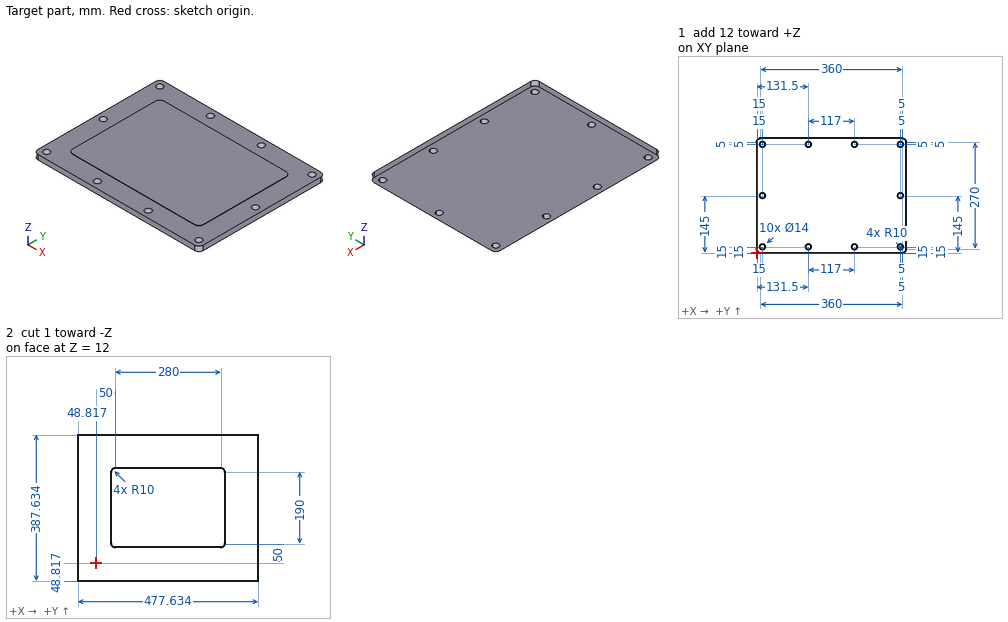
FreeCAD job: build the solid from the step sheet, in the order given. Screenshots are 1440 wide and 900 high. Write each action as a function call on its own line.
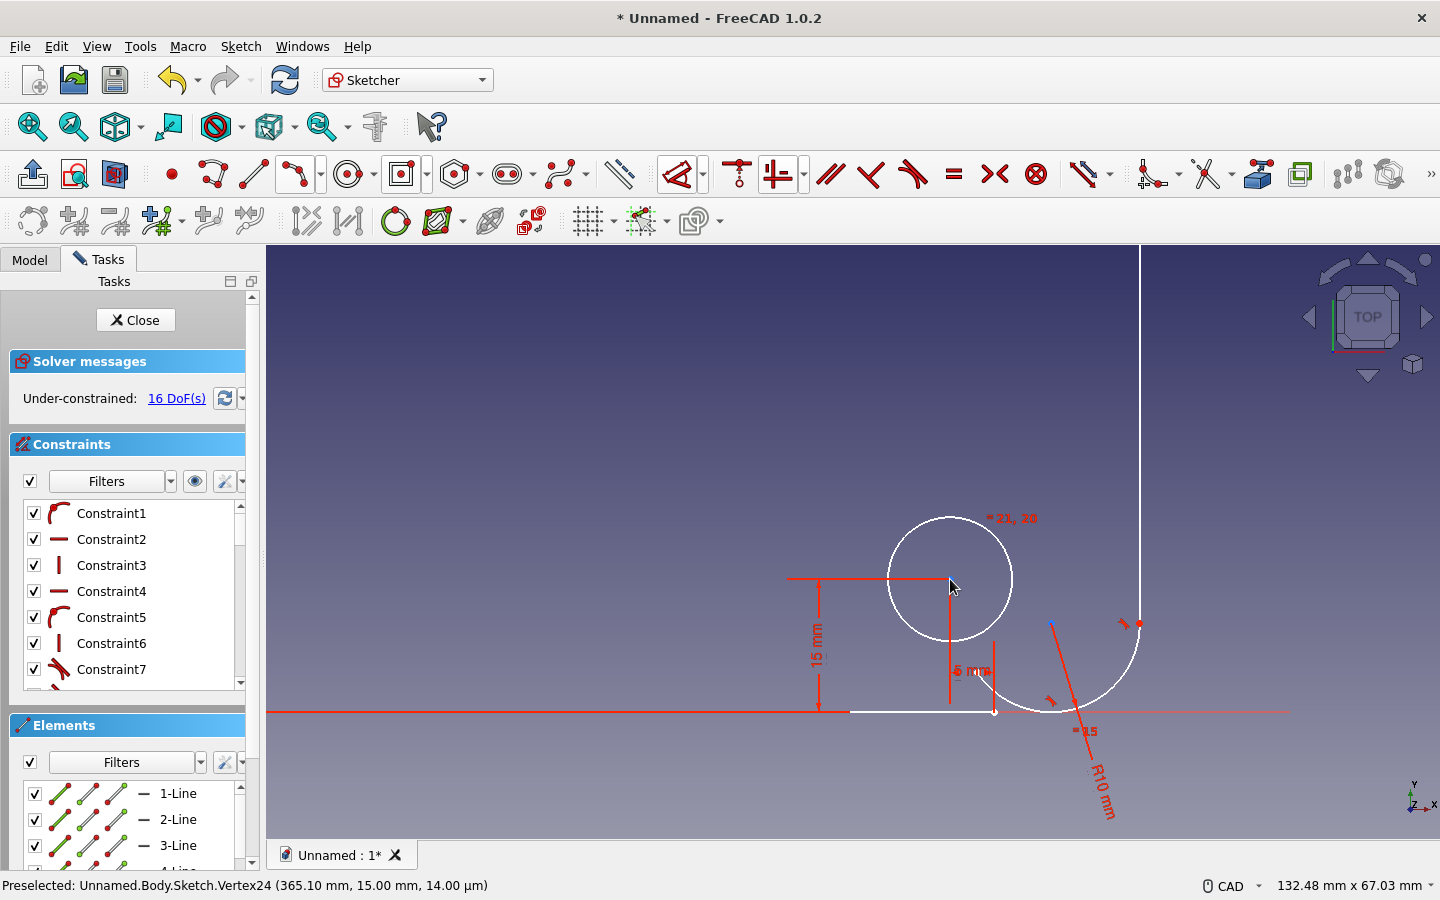
click(977, 673)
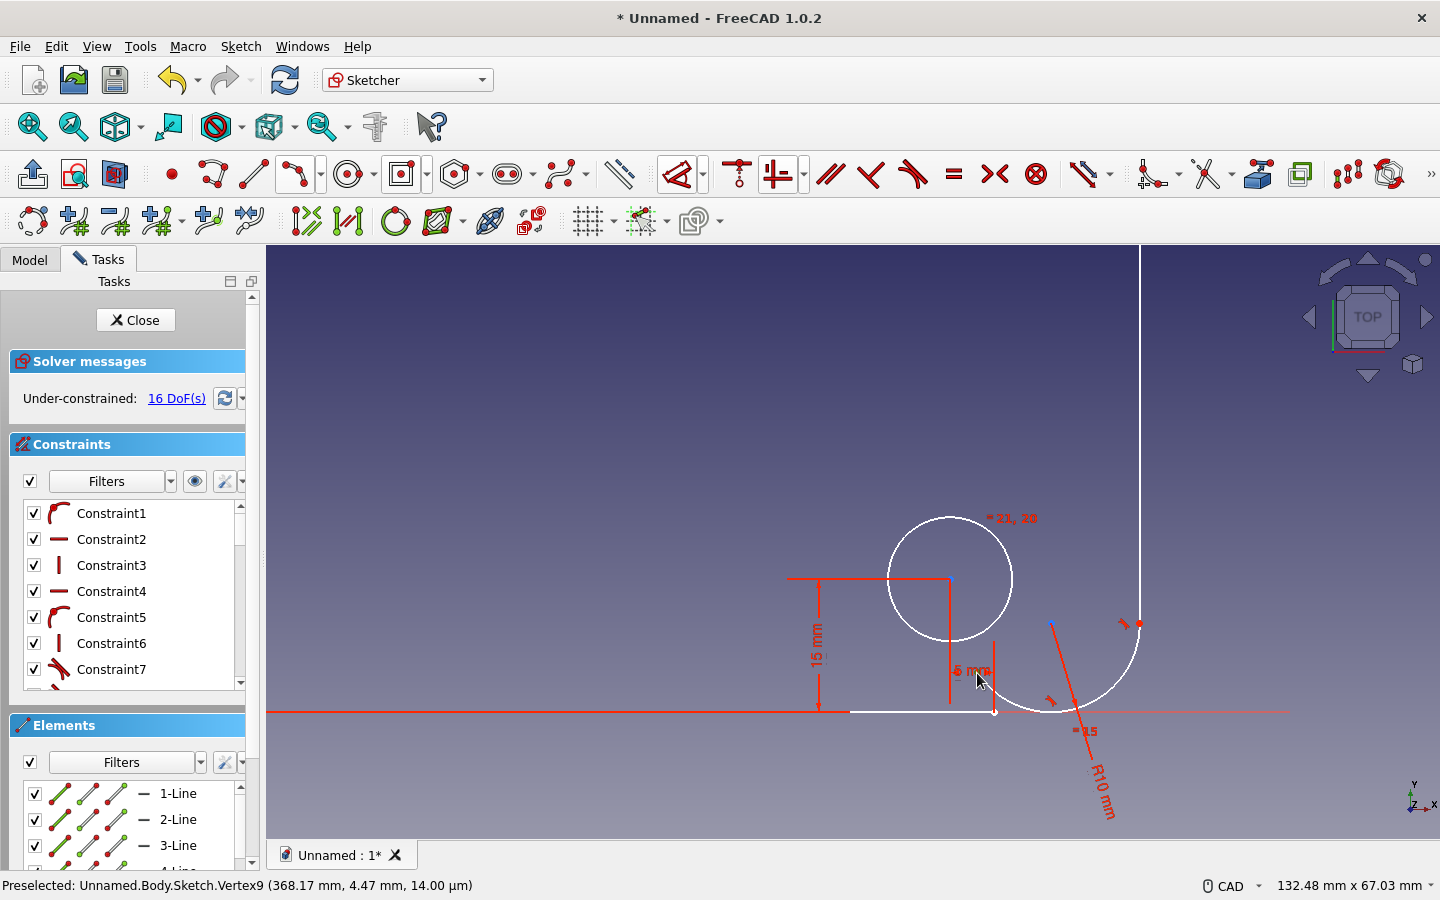
click(950, 579)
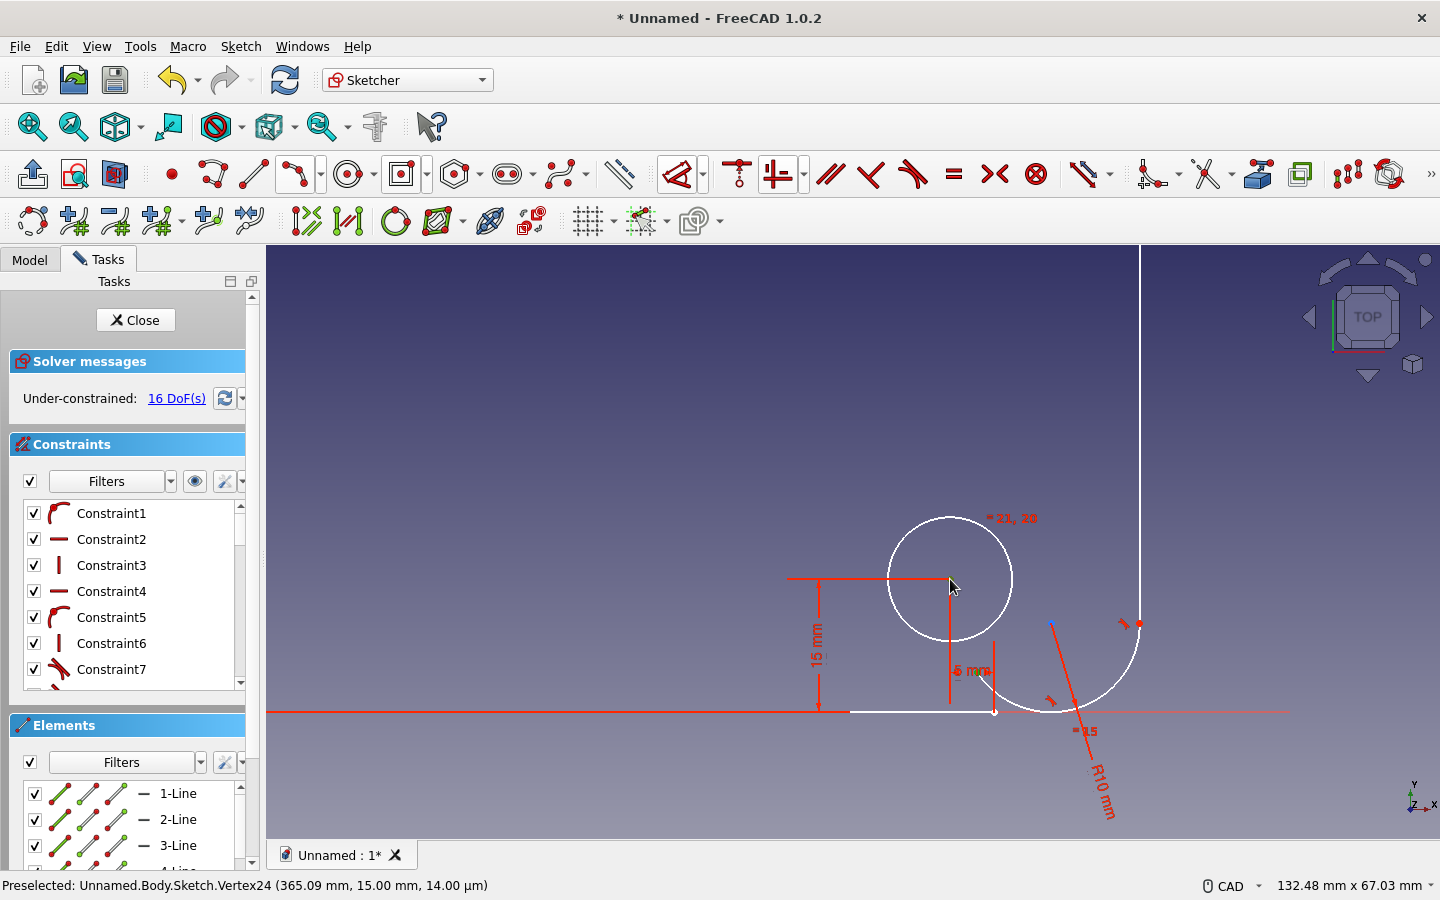
click(702, 174)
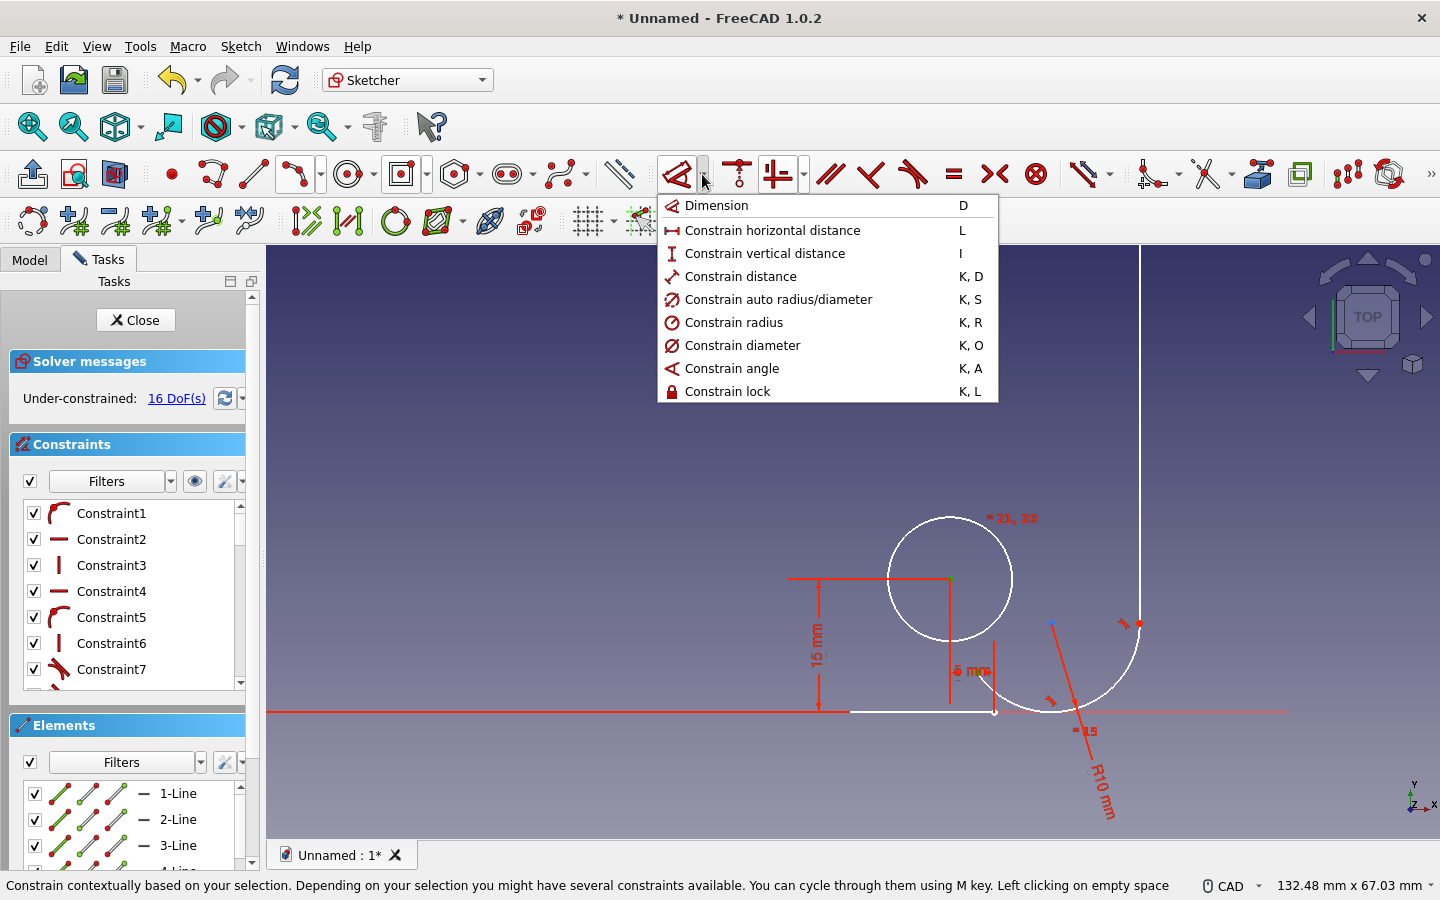
click(828, 230)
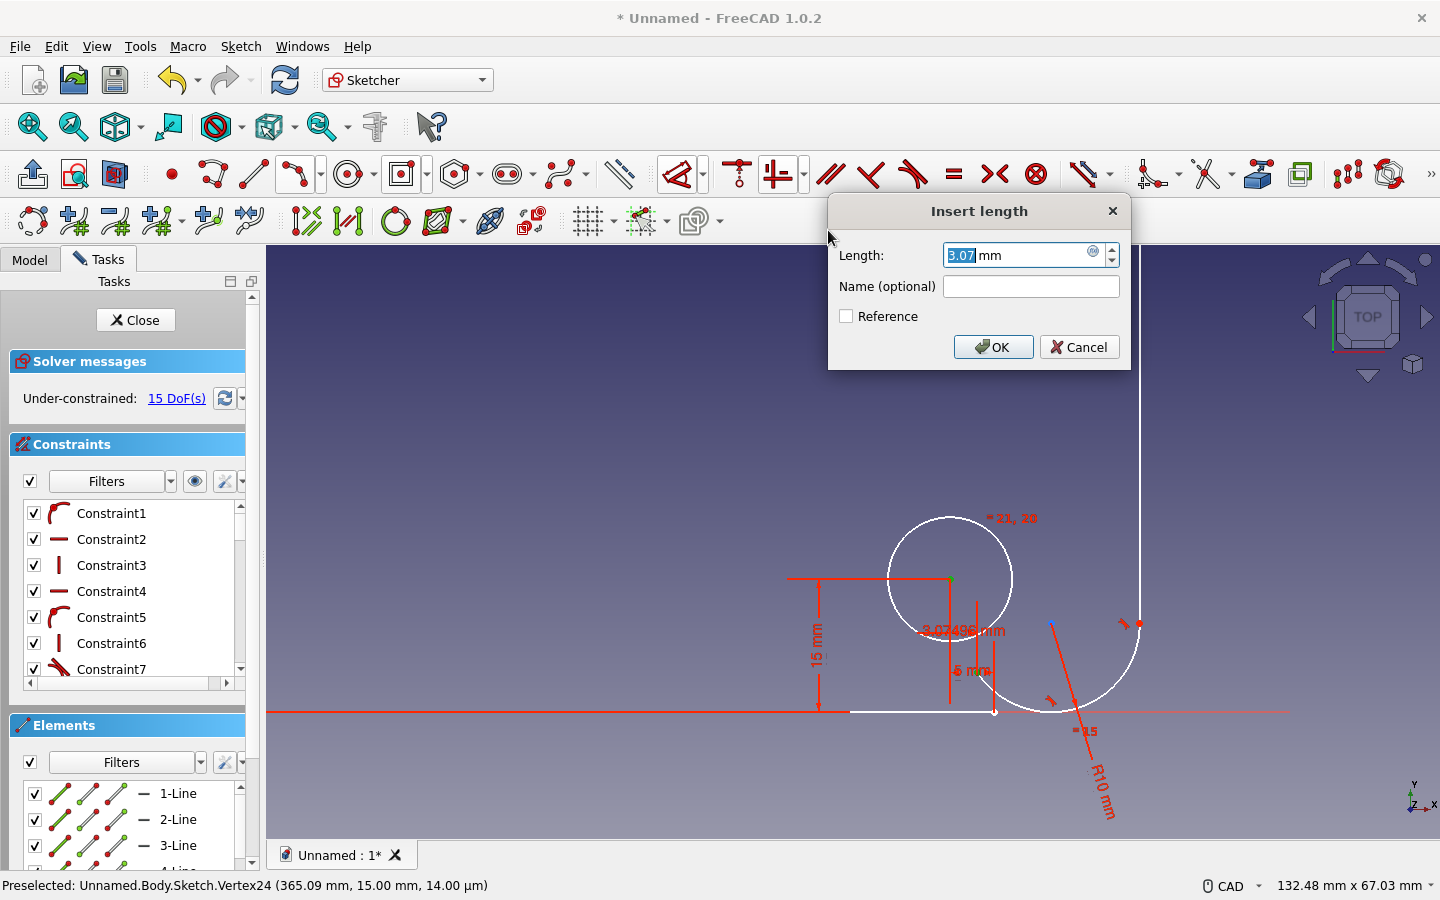
text(5)
key(Return)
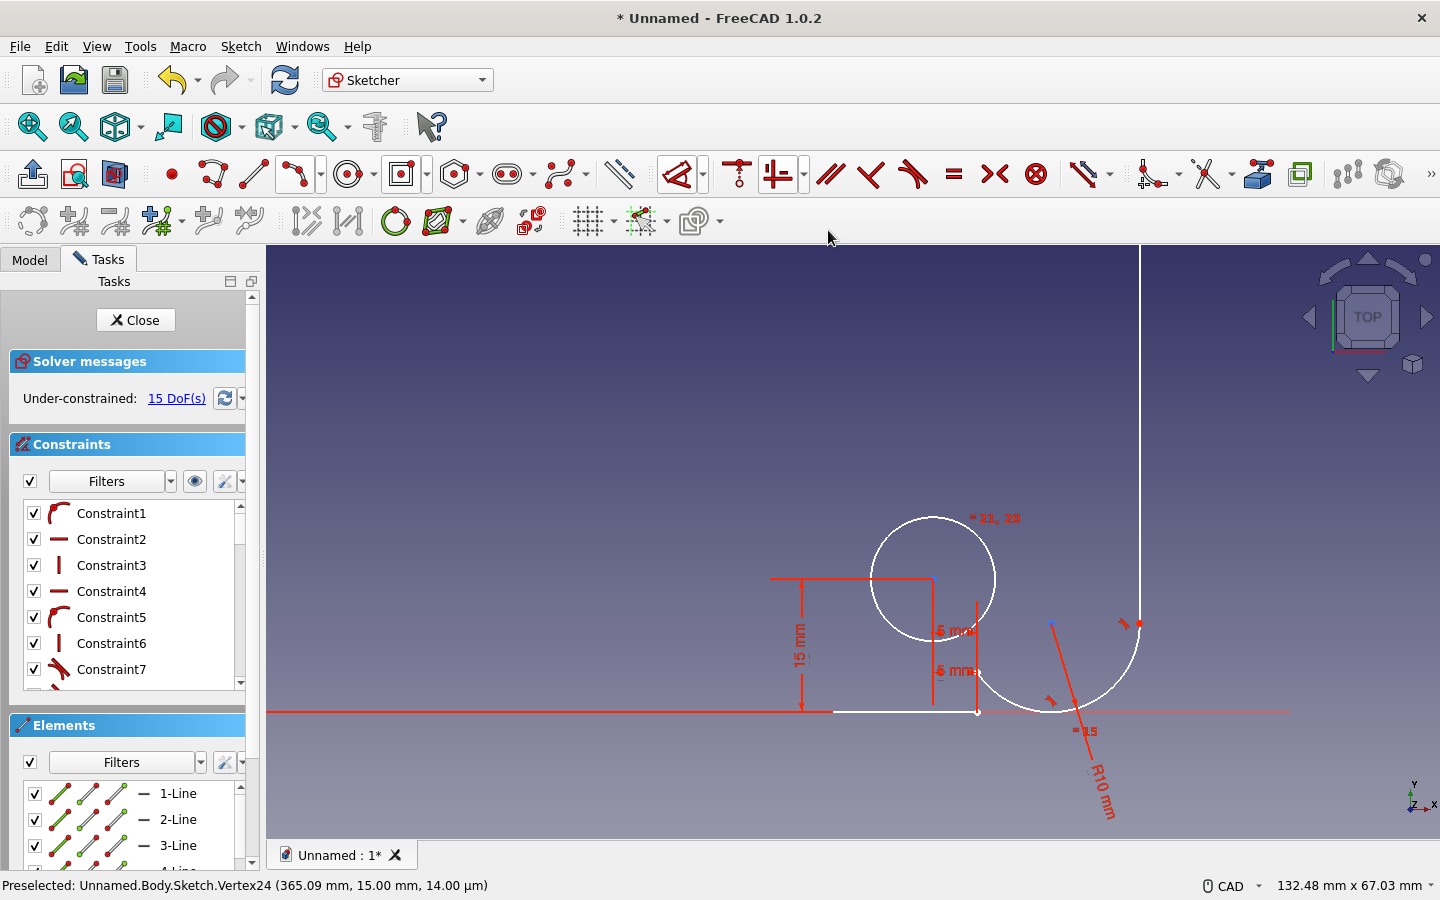
scroll(1001, 716, down, 10)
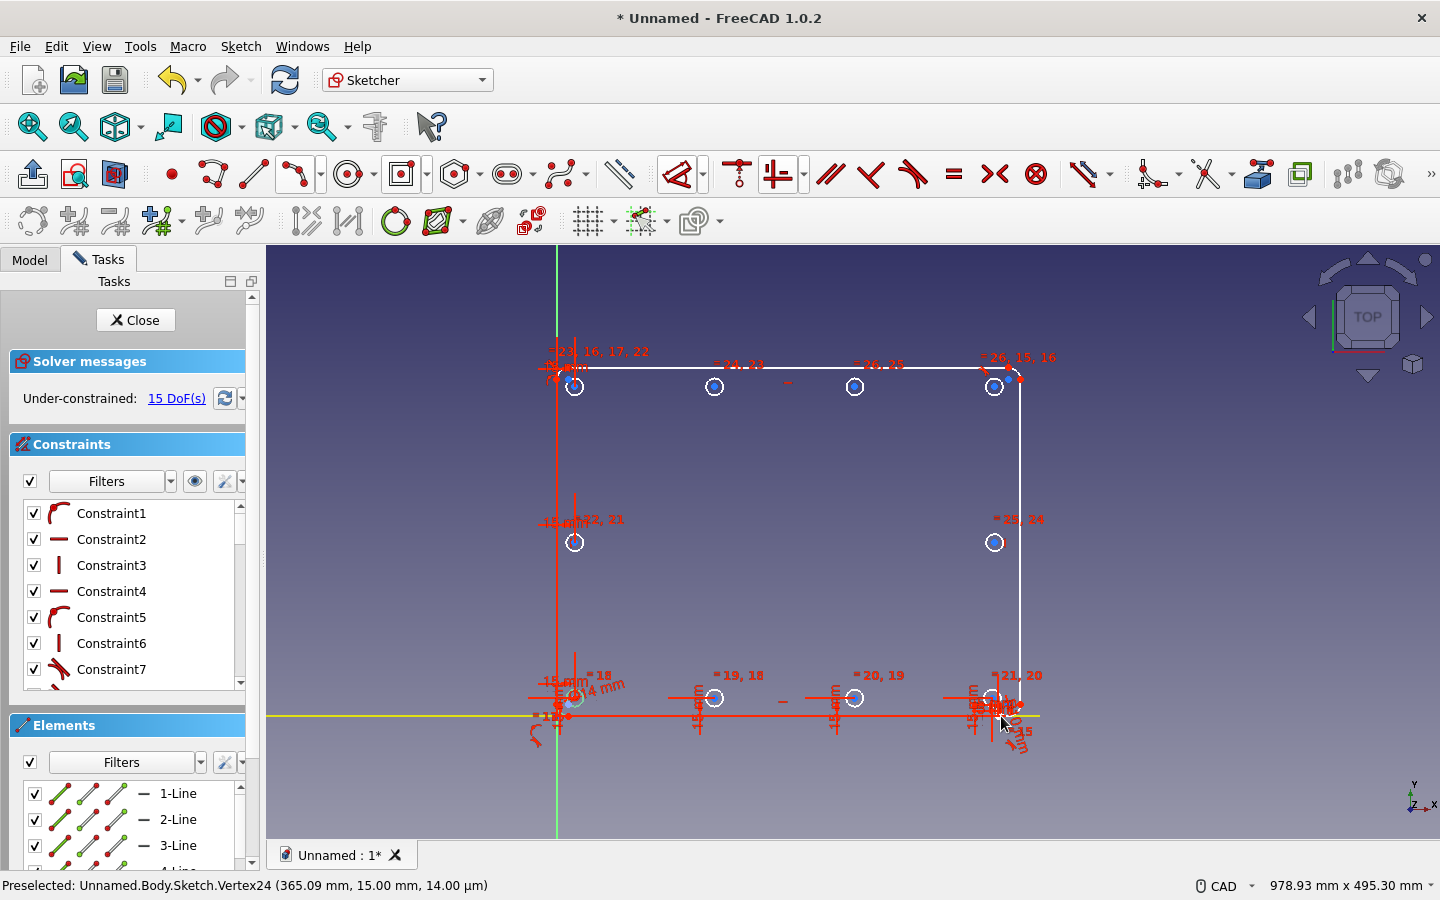
scroll(557, 380, up, 10)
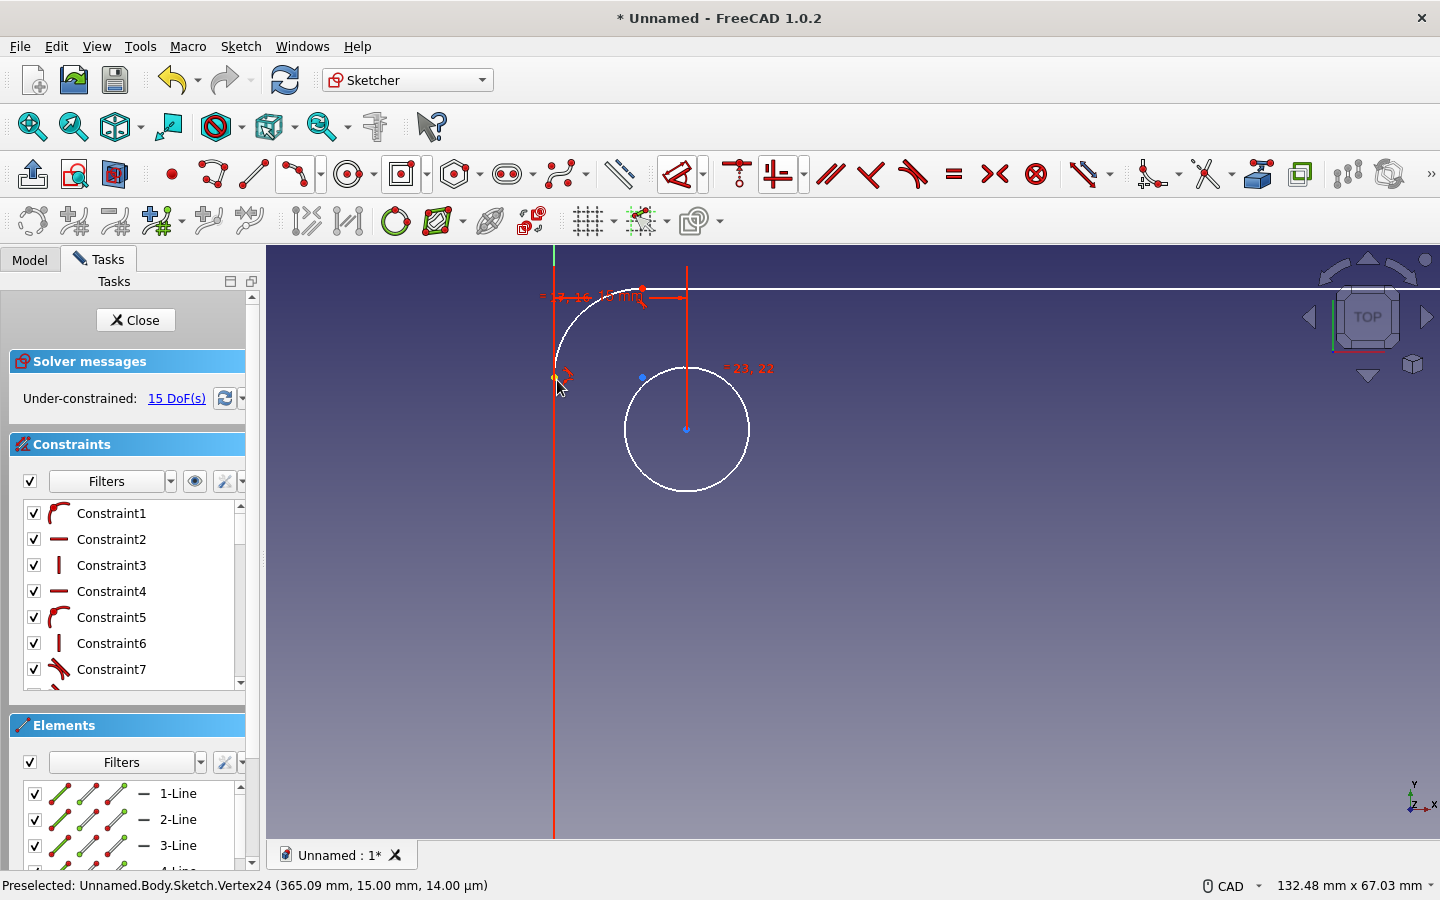
click(554, 377)